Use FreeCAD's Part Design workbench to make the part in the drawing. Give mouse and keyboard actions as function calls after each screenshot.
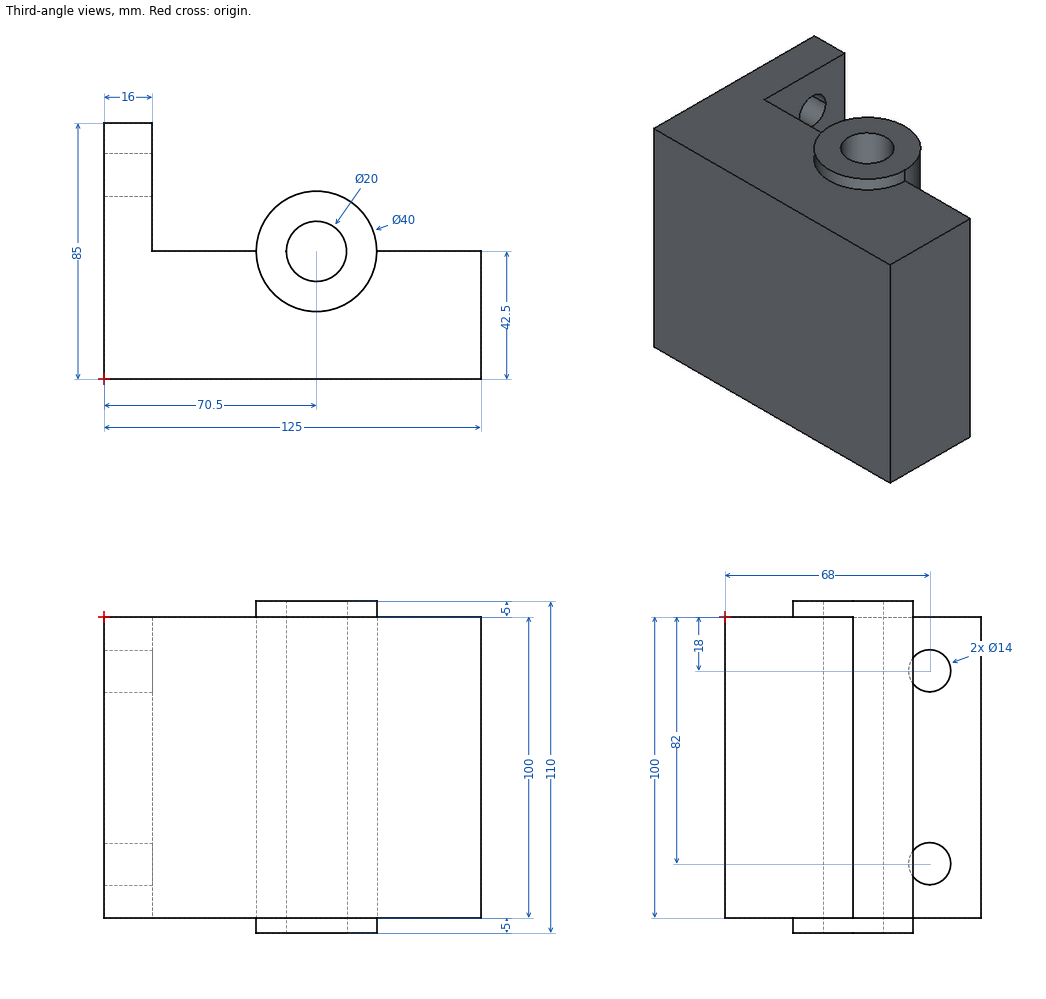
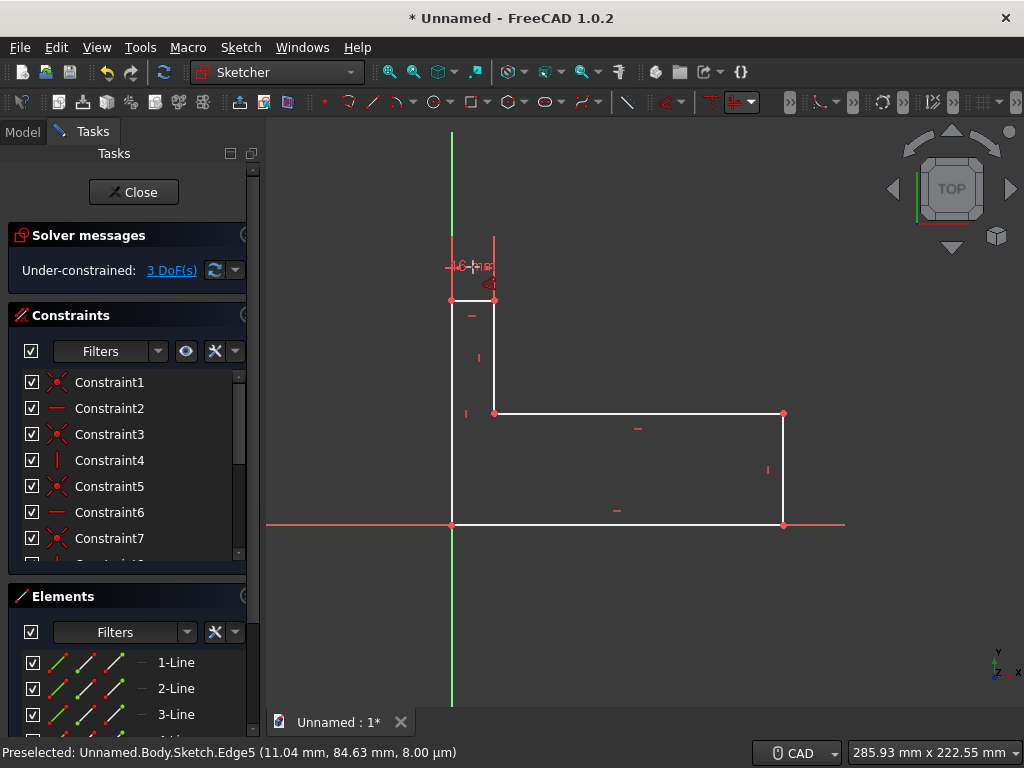
click(452, 368)
click(418, 413)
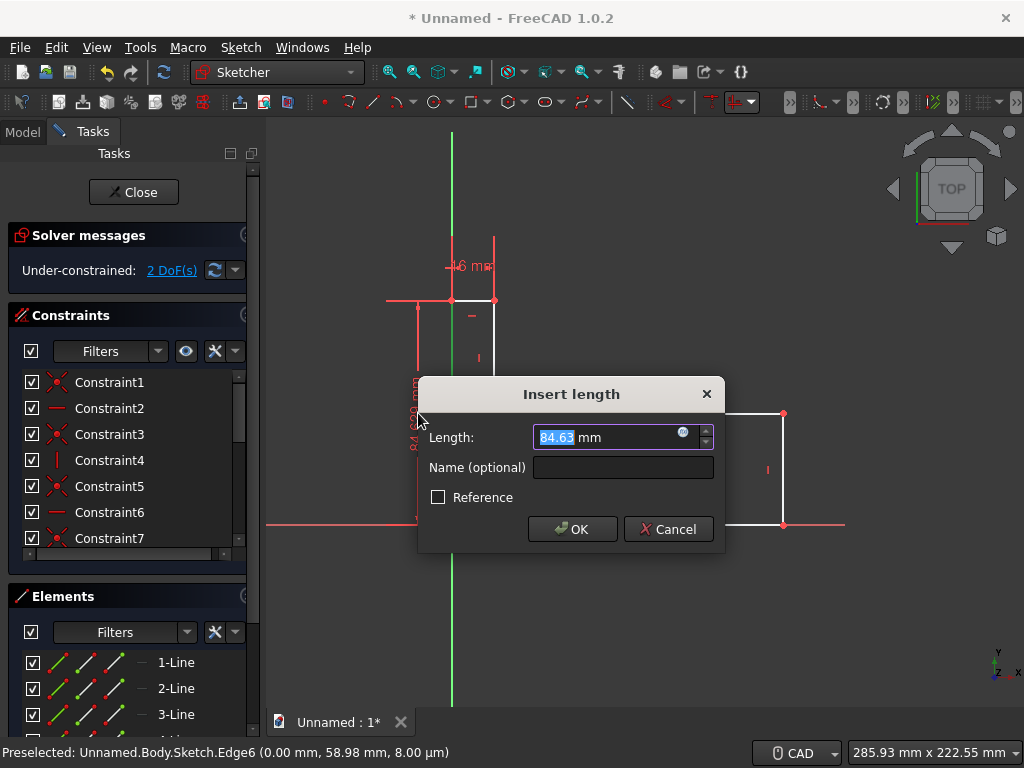
text(85)
key(Return)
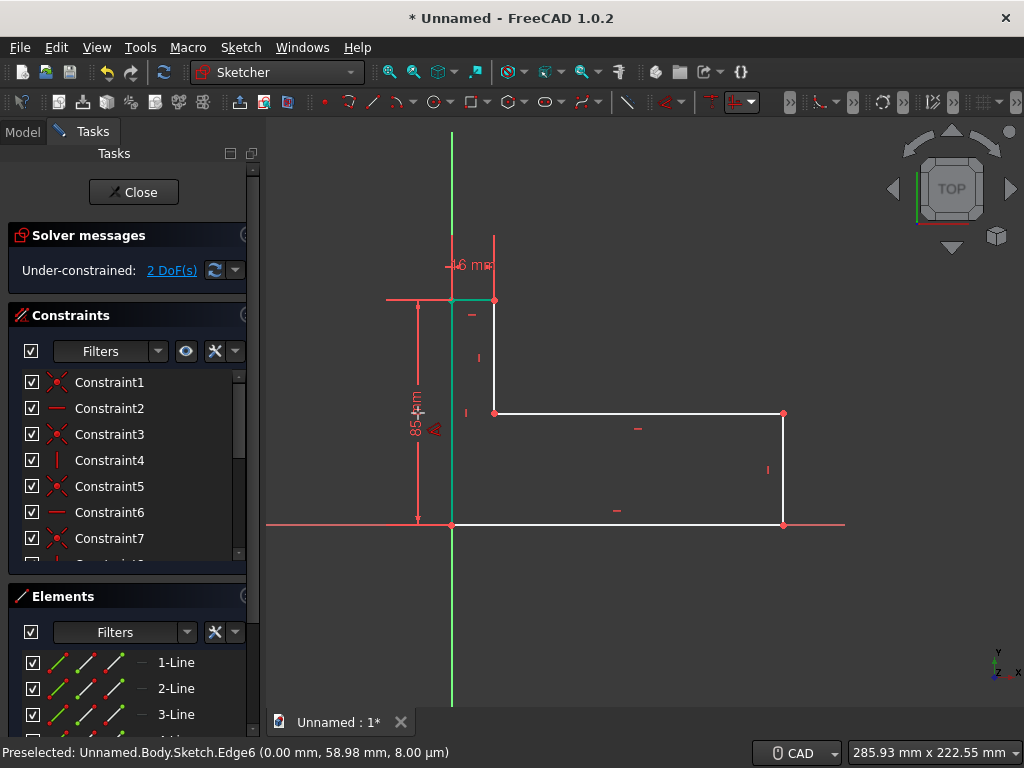
click(551, 525)
click(617, 559)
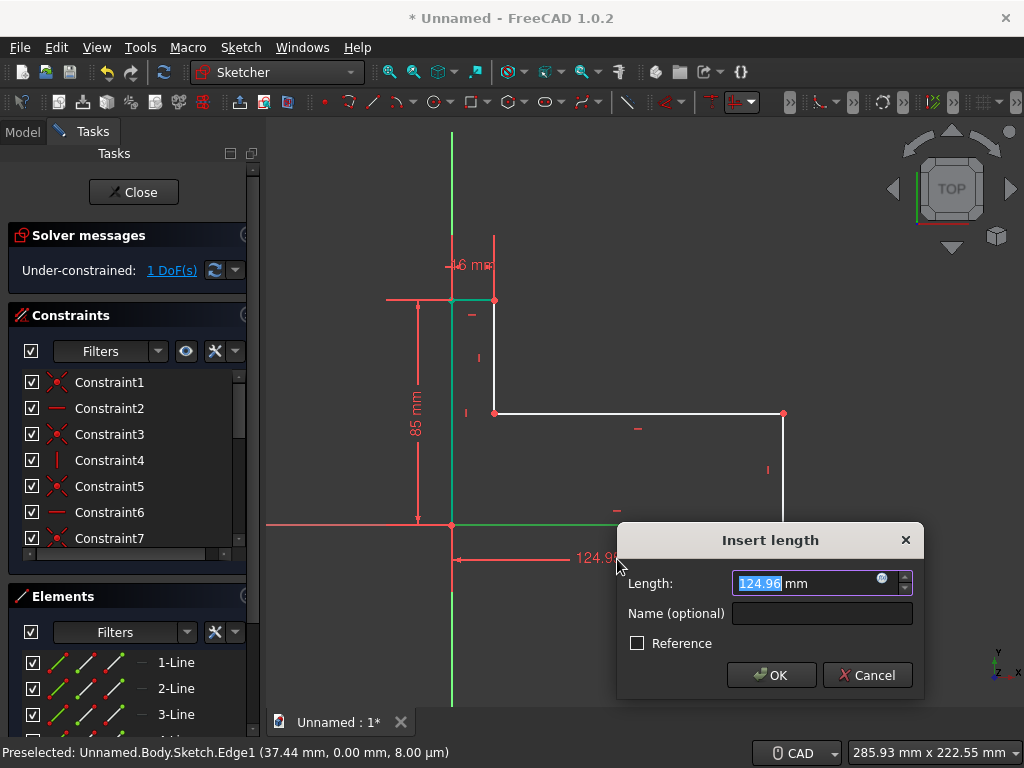
text(125)
key(Return)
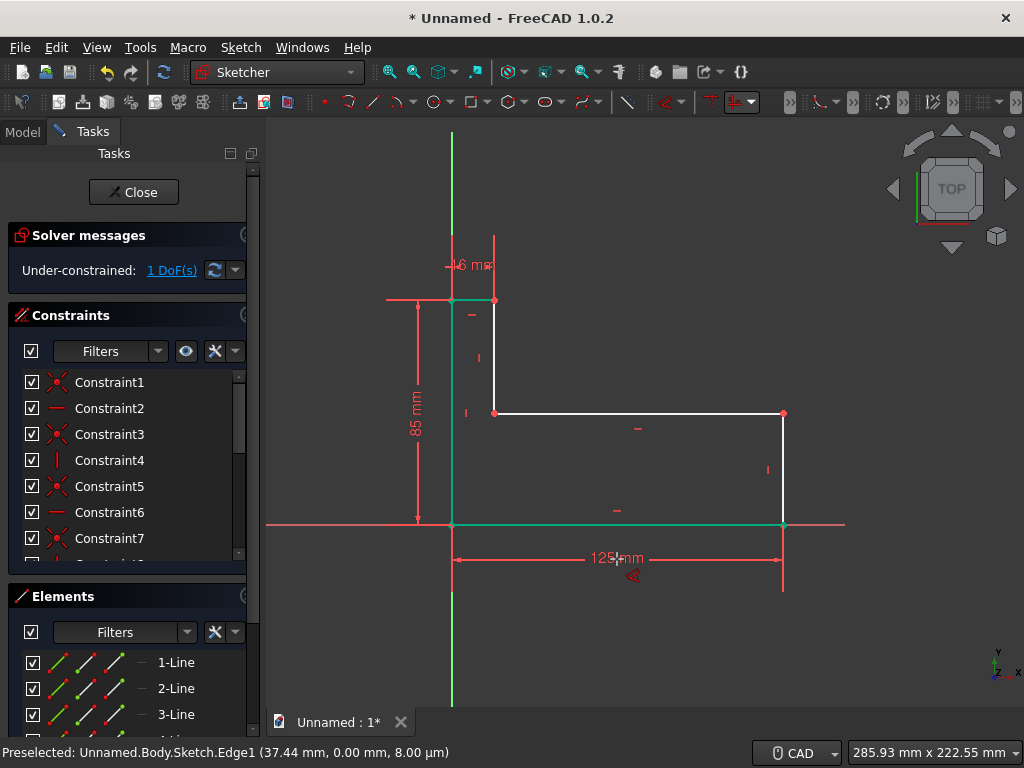
click(783, 492)
click(817, 470)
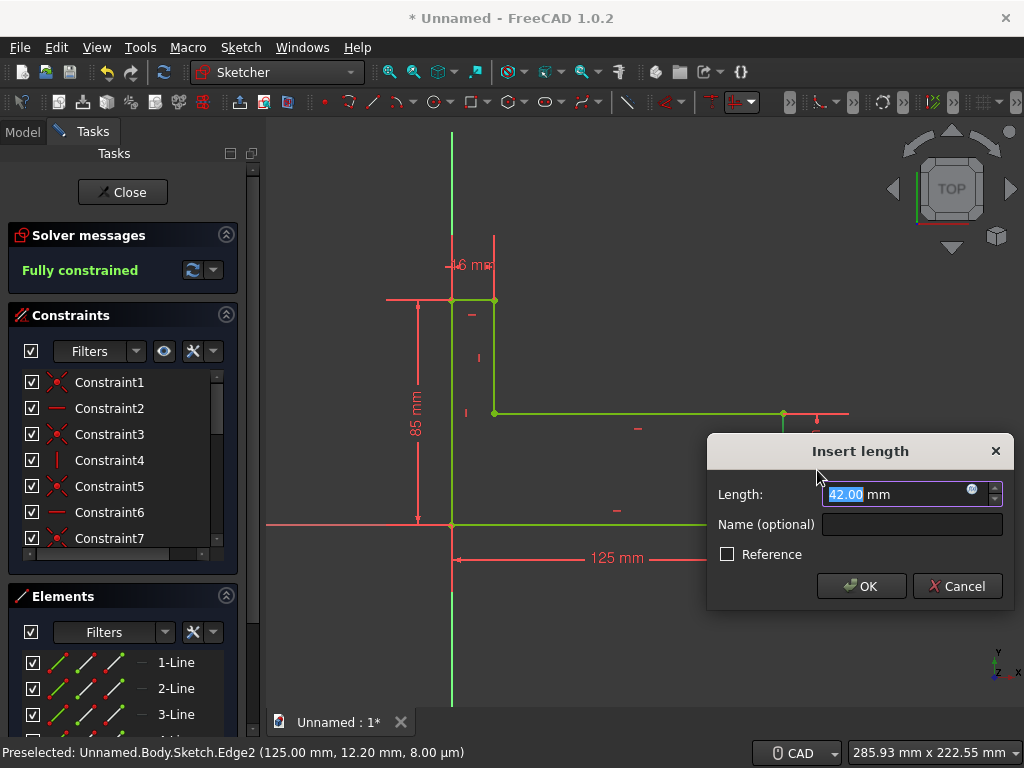
text(42.5)
key(Return)
key(Escape)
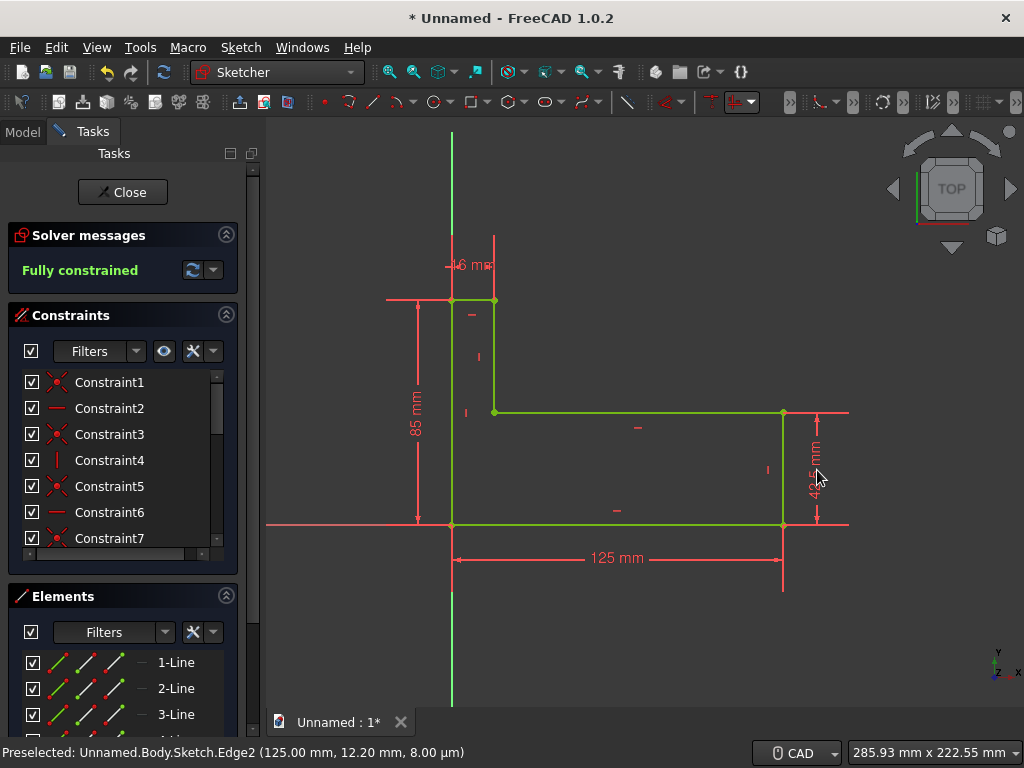
click(123, 192)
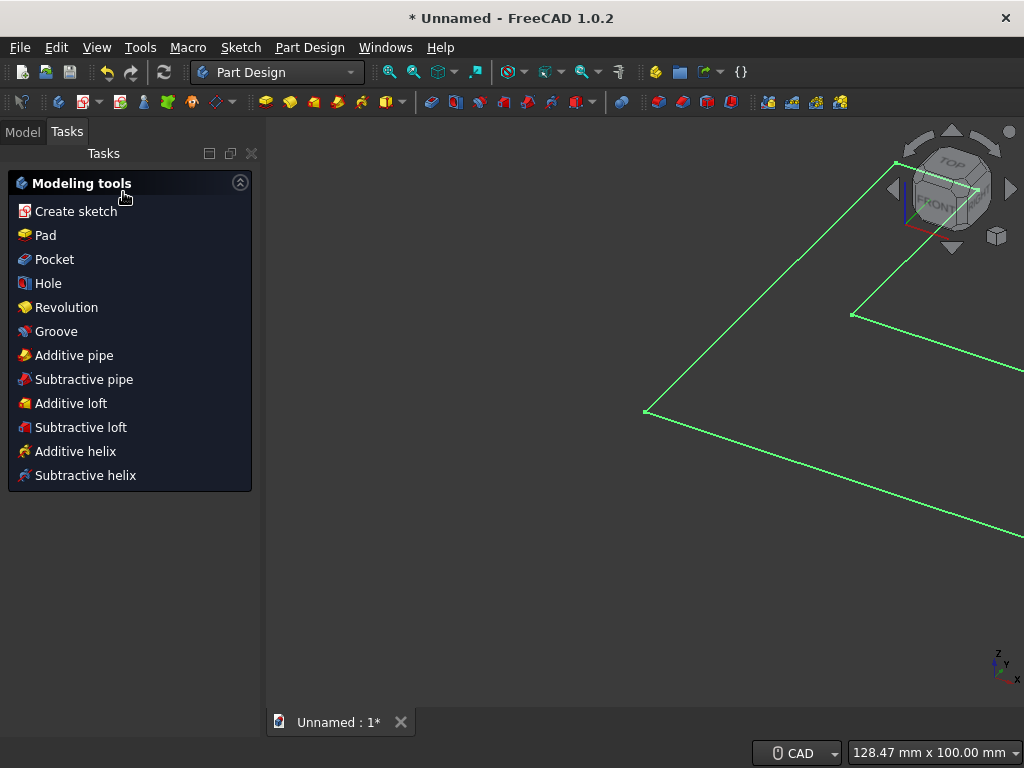
click(266, 102)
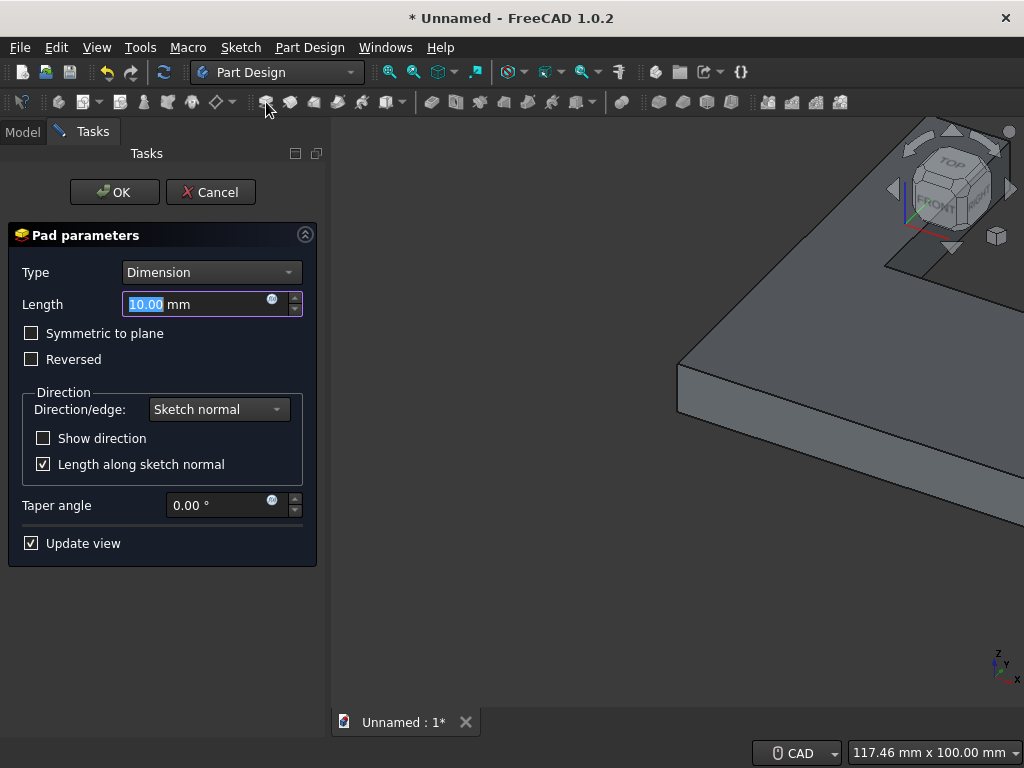
text(100)
key(Tab)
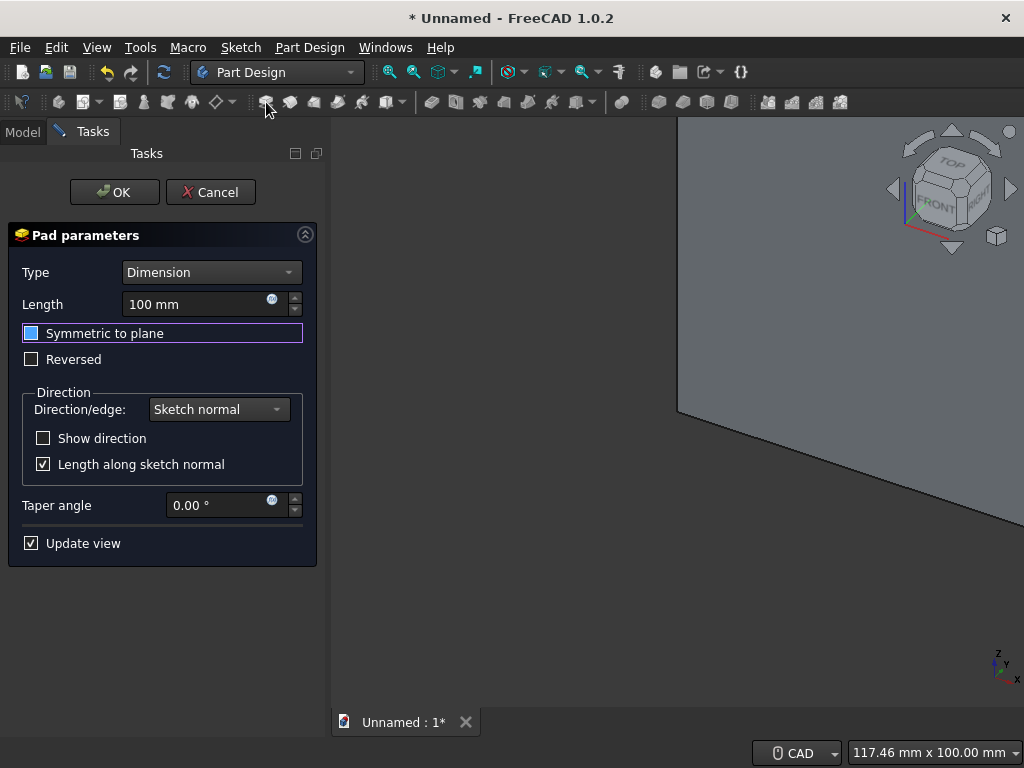
click(30, 359)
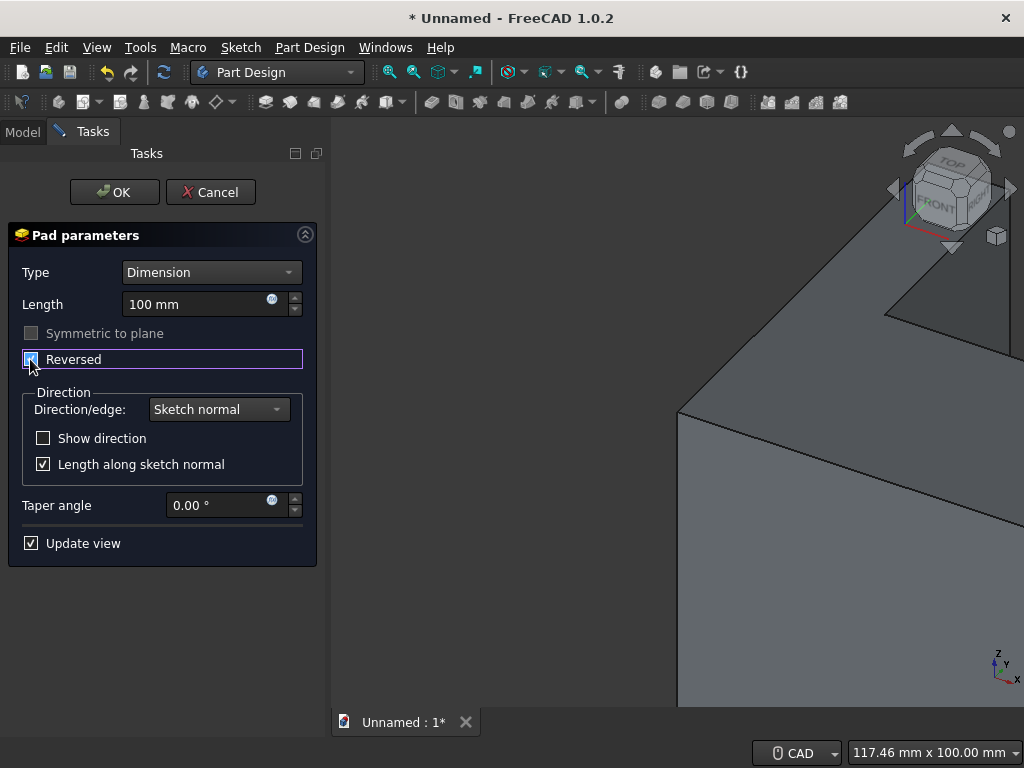
click(115, 192)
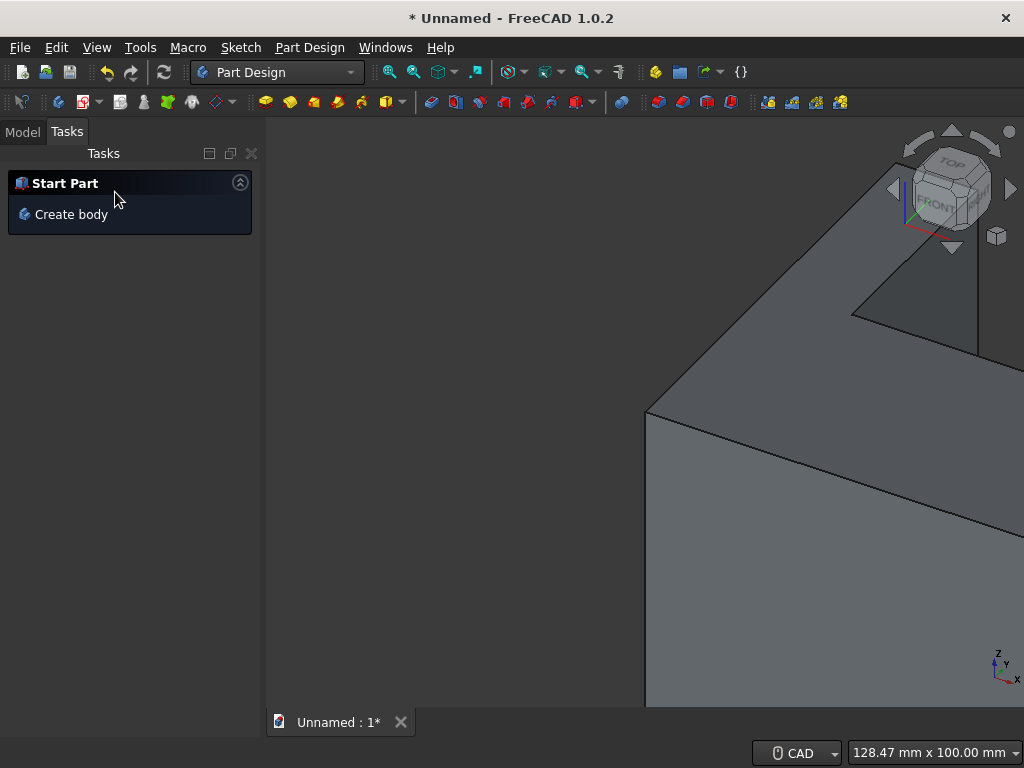
click(390, 72)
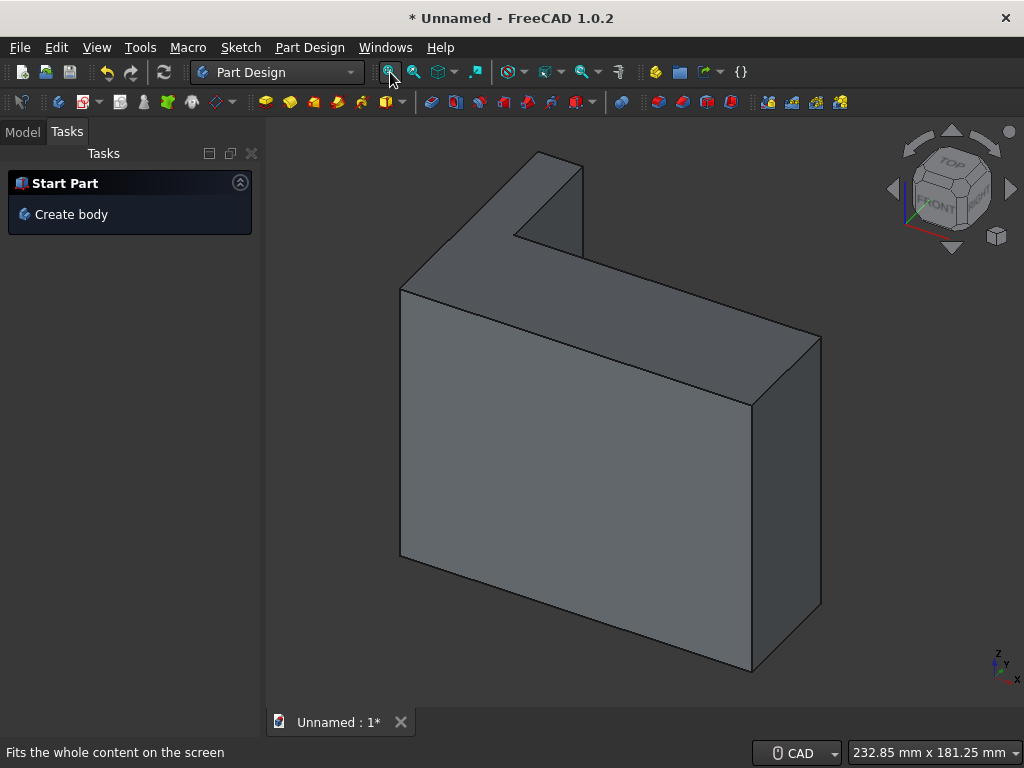
key(0)